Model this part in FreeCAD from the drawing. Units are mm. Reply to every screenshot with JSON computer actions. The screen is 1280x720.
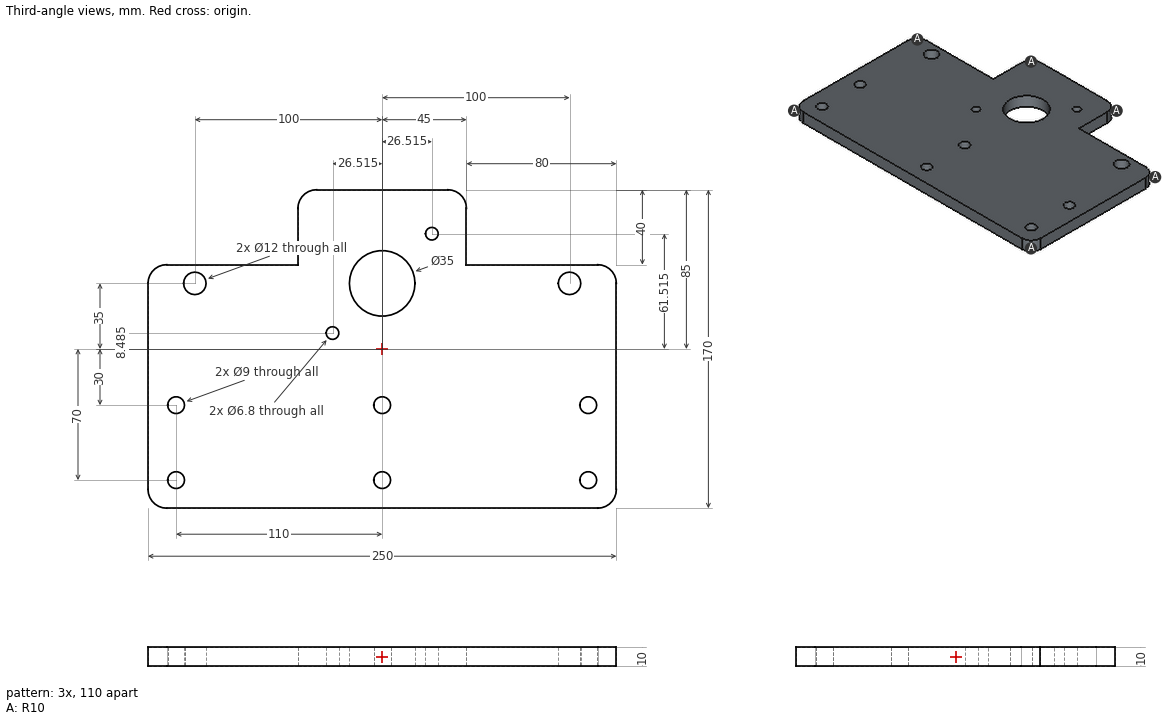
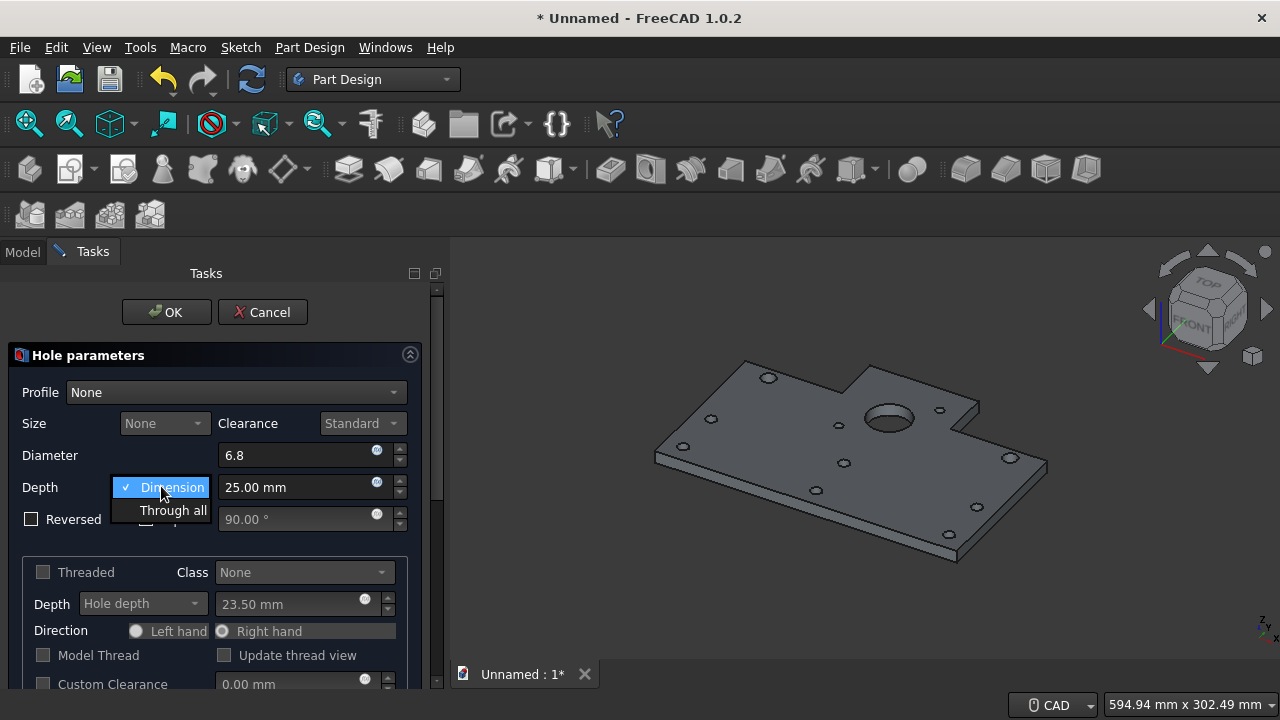
{"action": "left_click", "coordinate": [160, 510]}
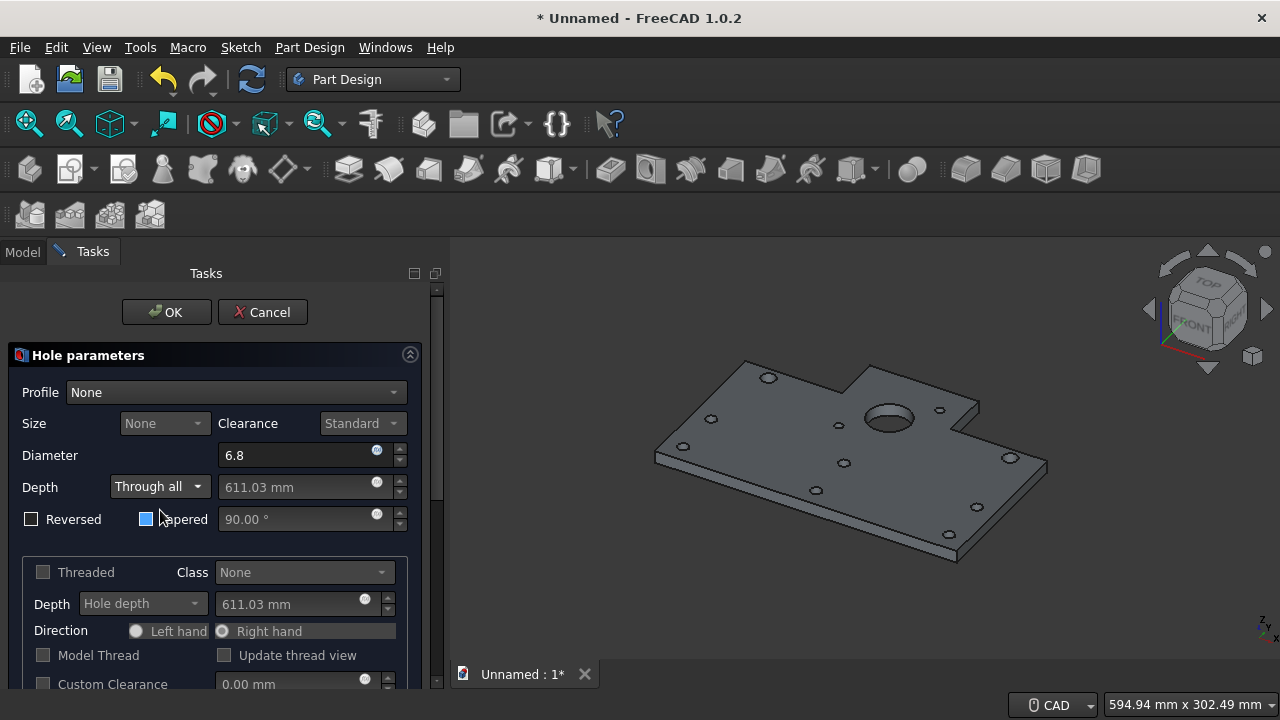
{"action": "left_click", "coordinate": [167, 312]}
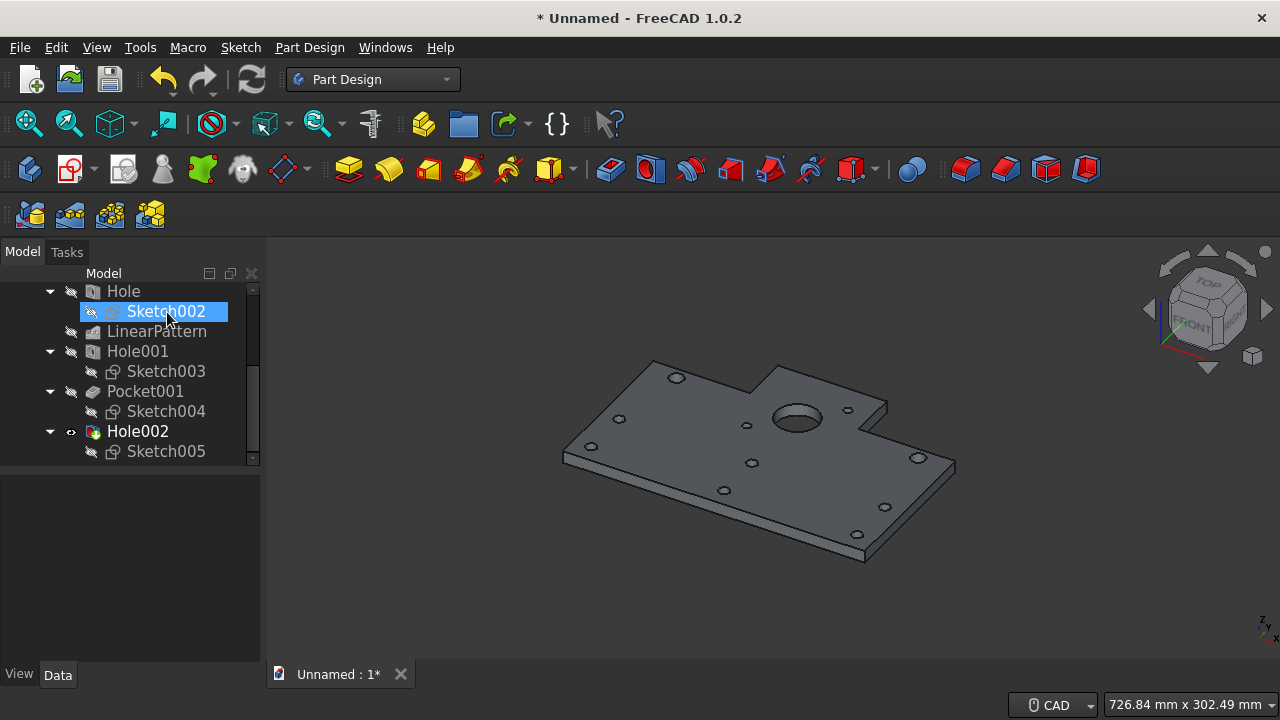
{"action": "left_click", "coordinate": [865, 557]}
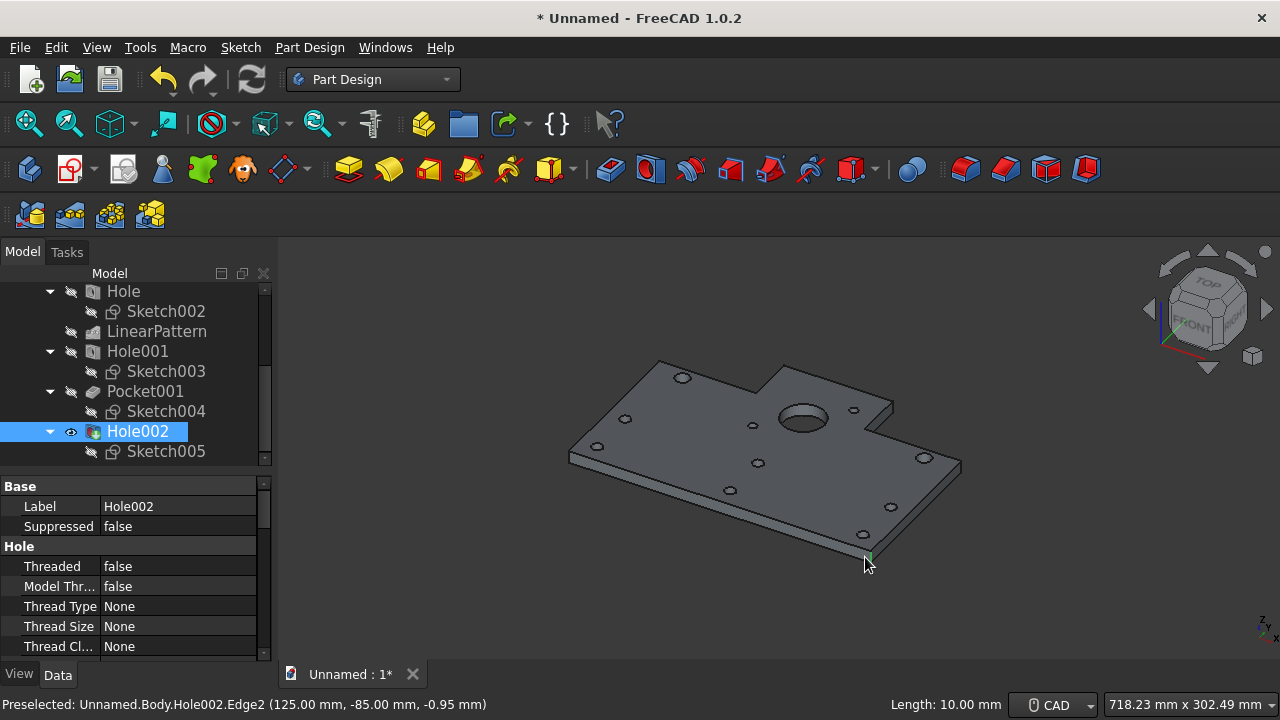
{"action": "scroll", "coordinate": [893, 406], "scroll_direction": "up", "scroll_amount": 6}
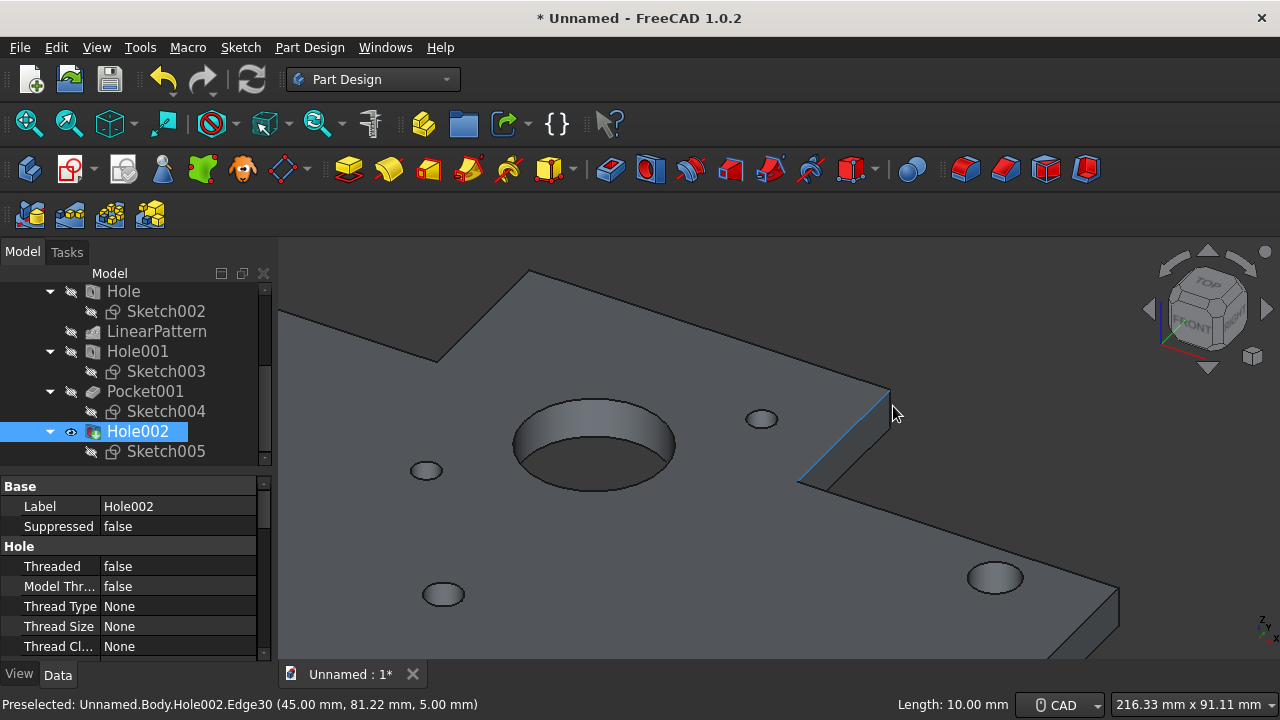
{"action": "left_click", "coordinate": [30, 124]}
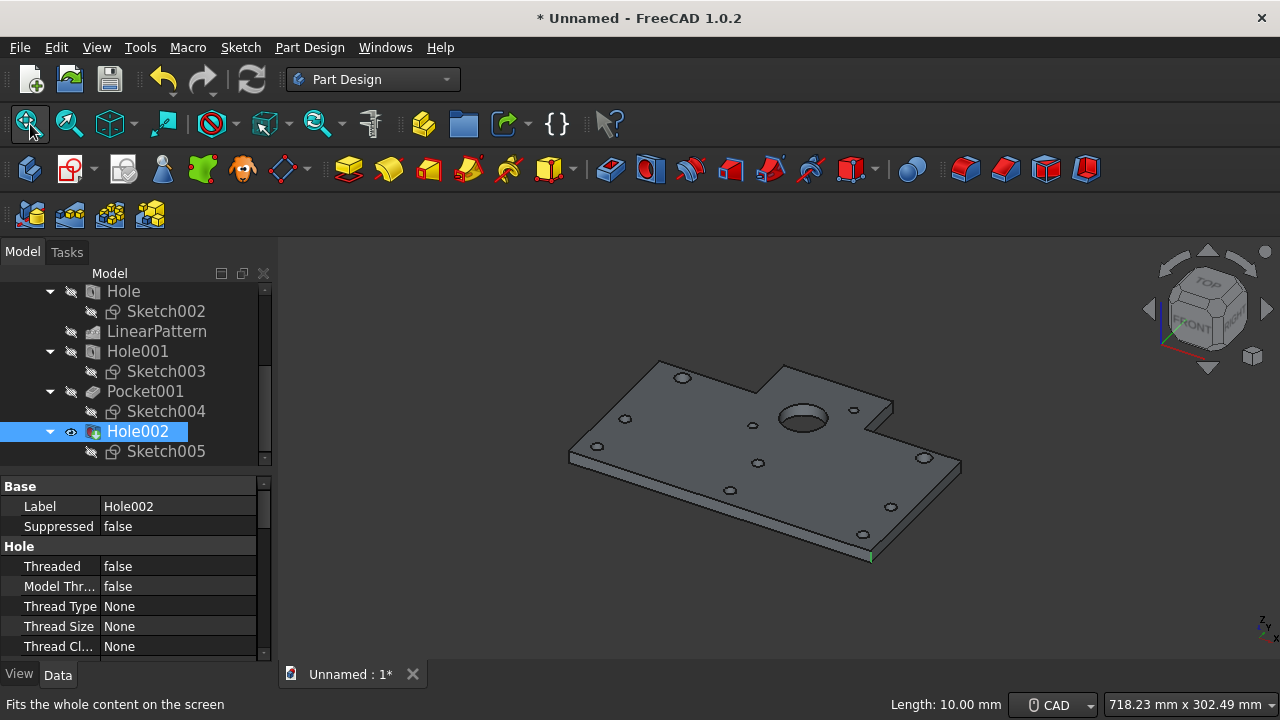
{"action": "key", "text": "0"}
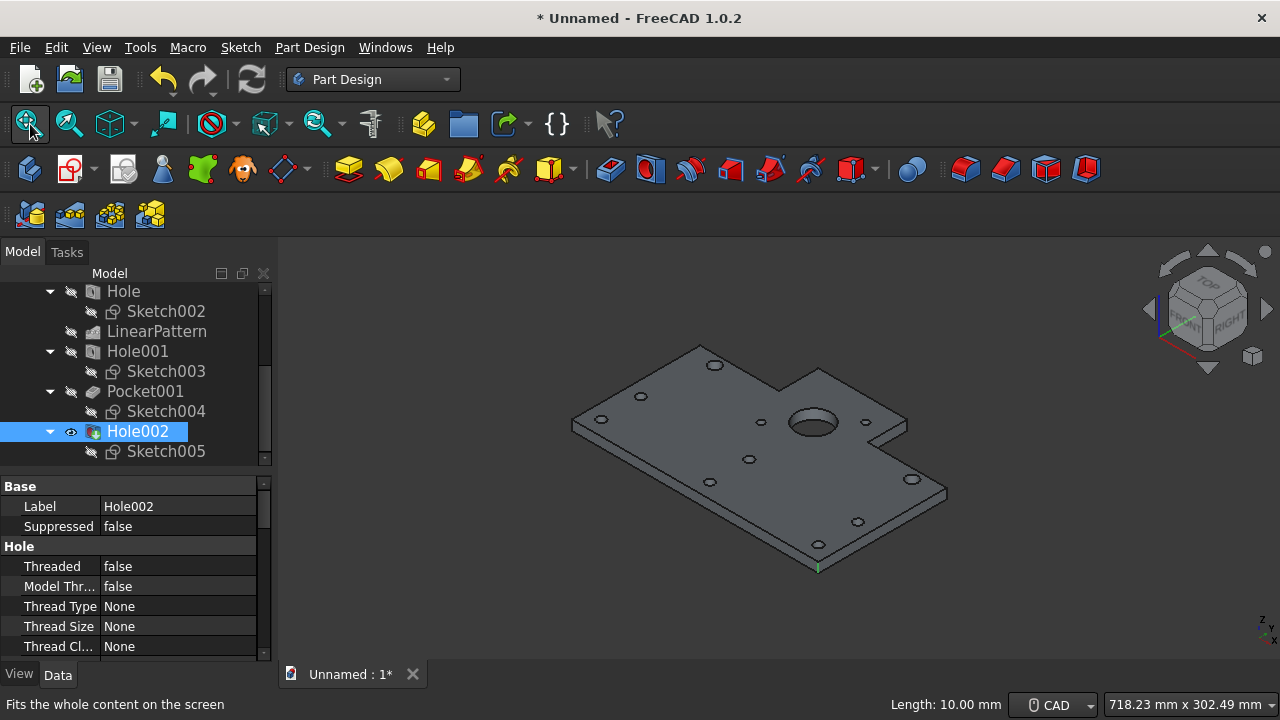
{"action": "scroll", "coordinate": [907, 424], "scroll_direction": "up", "scroll_amount": 6}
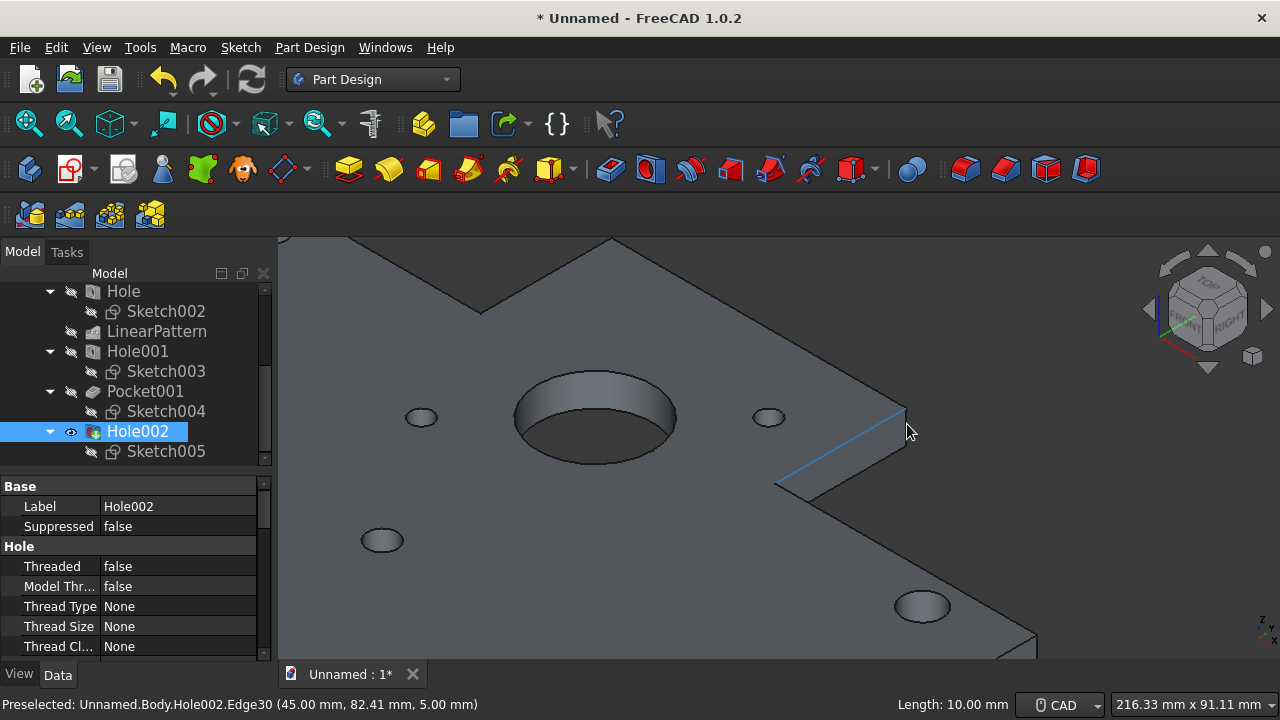
{"action": "left_click", "coordinate": [30, 124]}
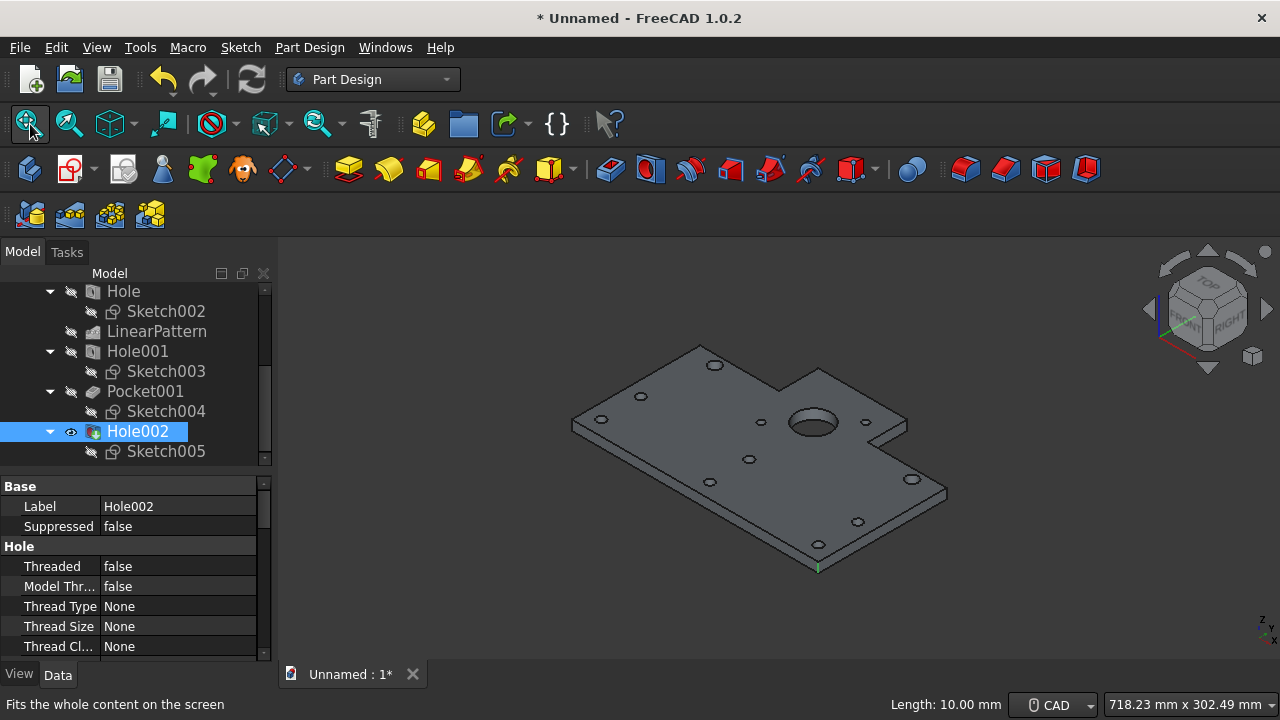
{"action": "key", "text": "2"}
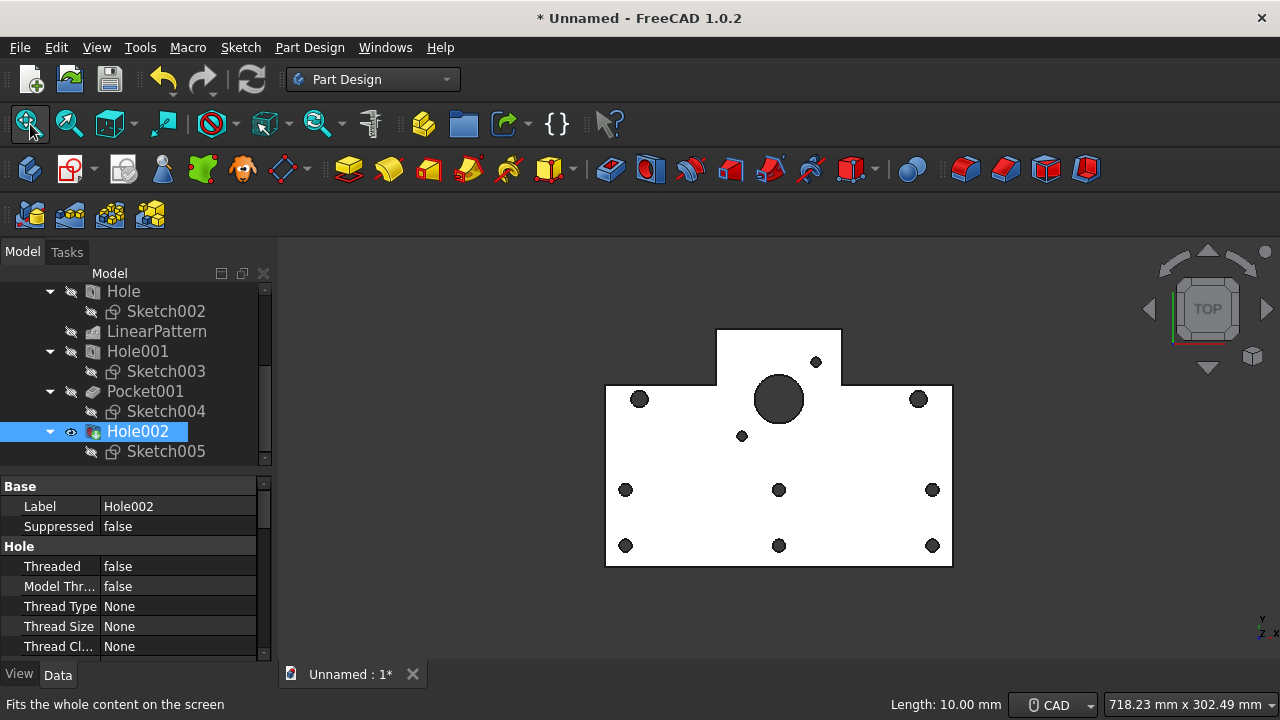
{"action": "scroll", "coordinate": [842, 328], "scroll_direction": "up", "scroll_amount": 6}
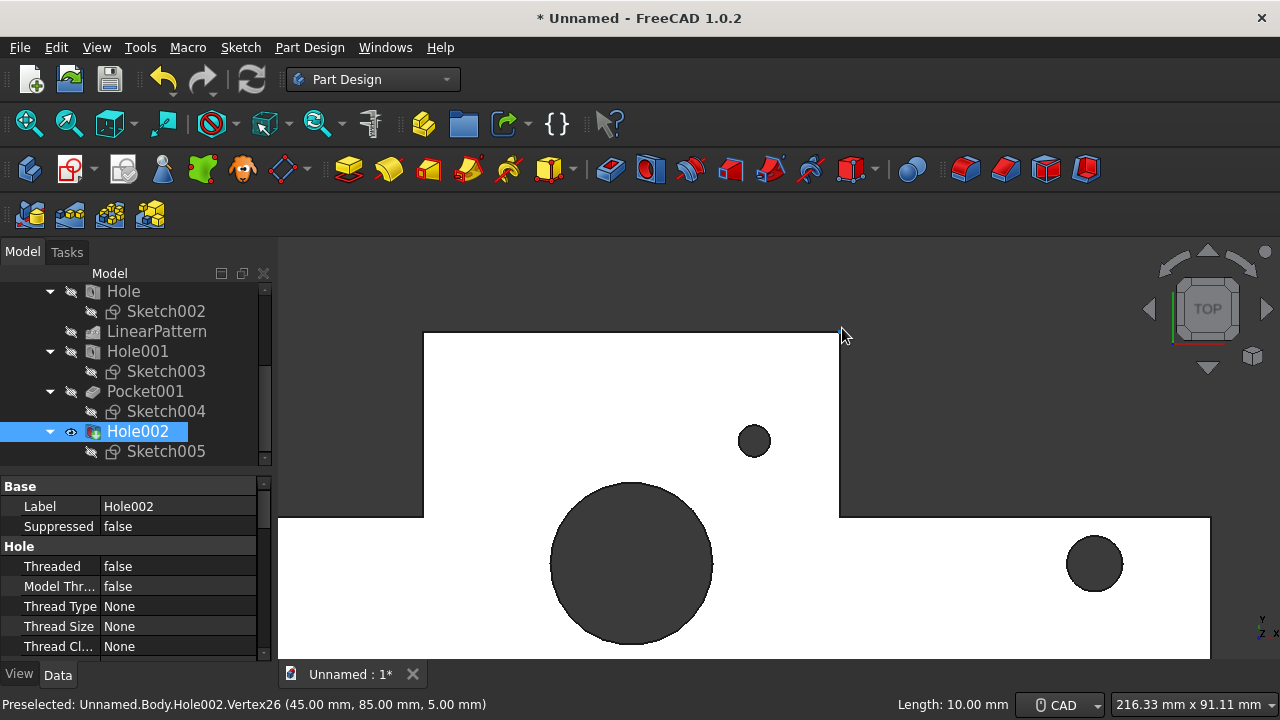
{"action": "left_click", "coordinate": [30, 124]}